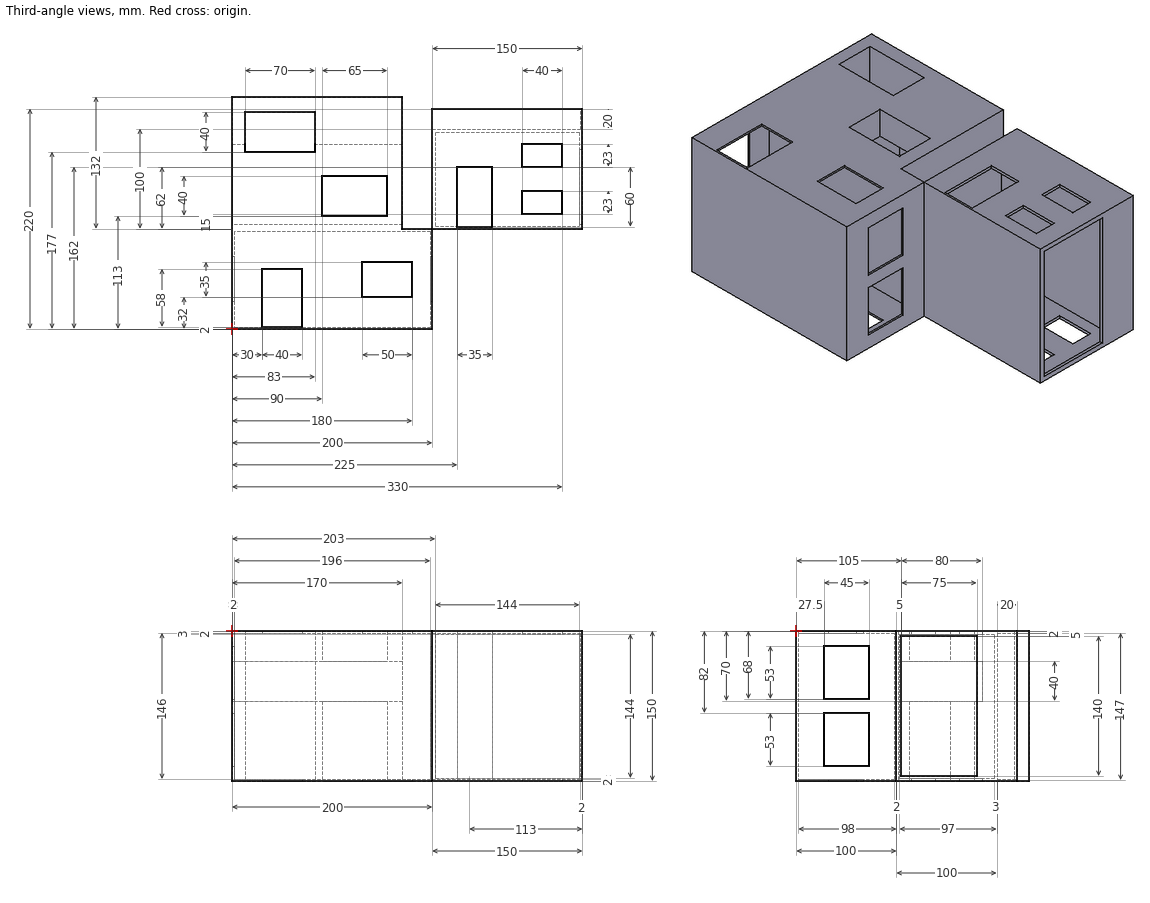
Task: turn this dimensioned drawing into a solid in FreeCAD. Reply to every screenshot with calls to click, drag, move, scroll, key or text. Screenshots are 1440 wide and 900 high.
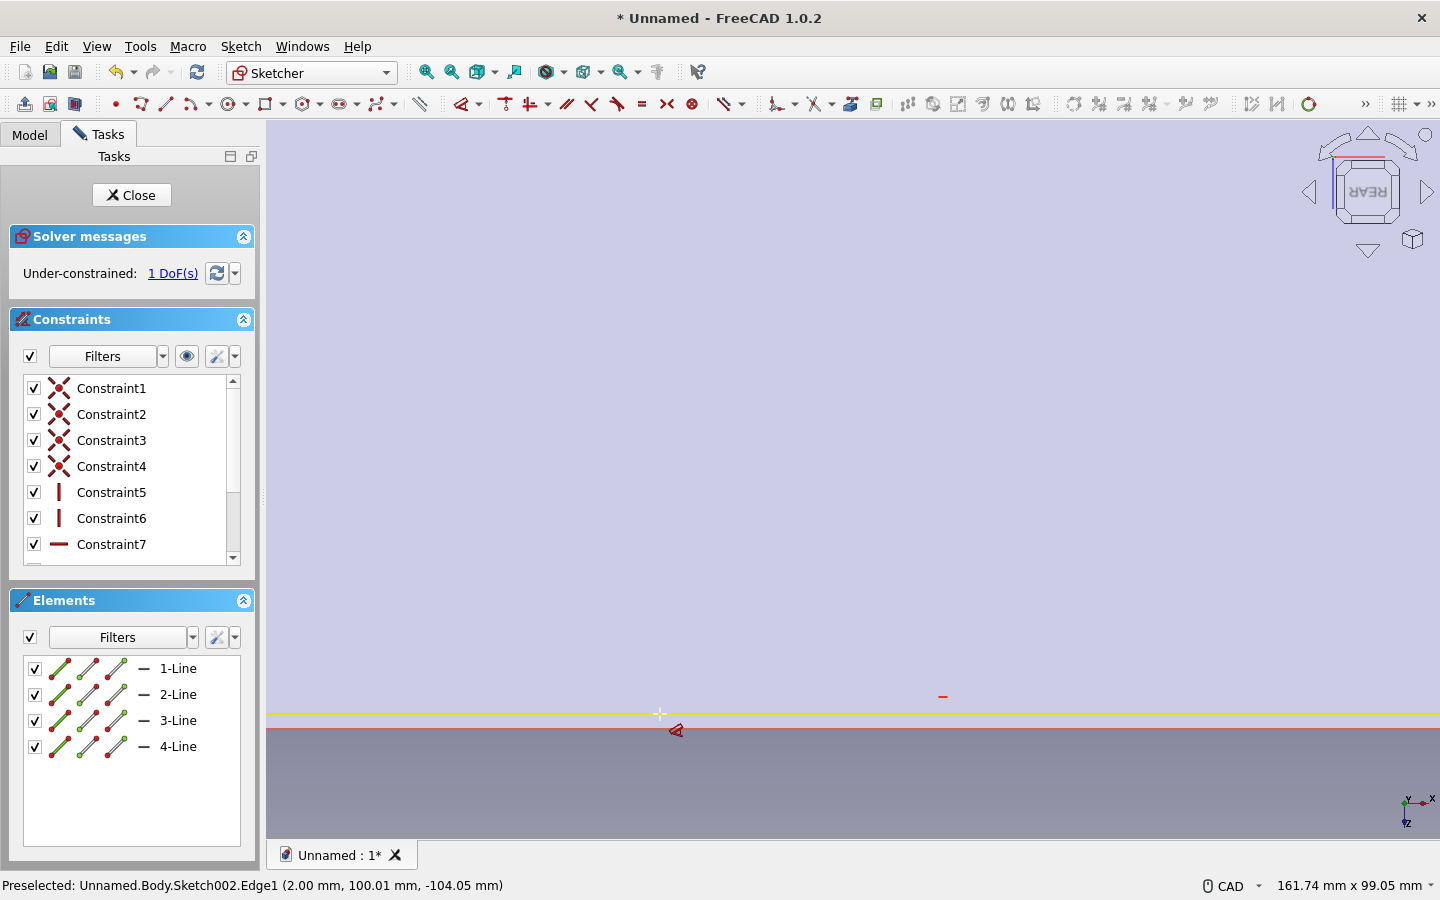
click(659, 714)
click(784, 748)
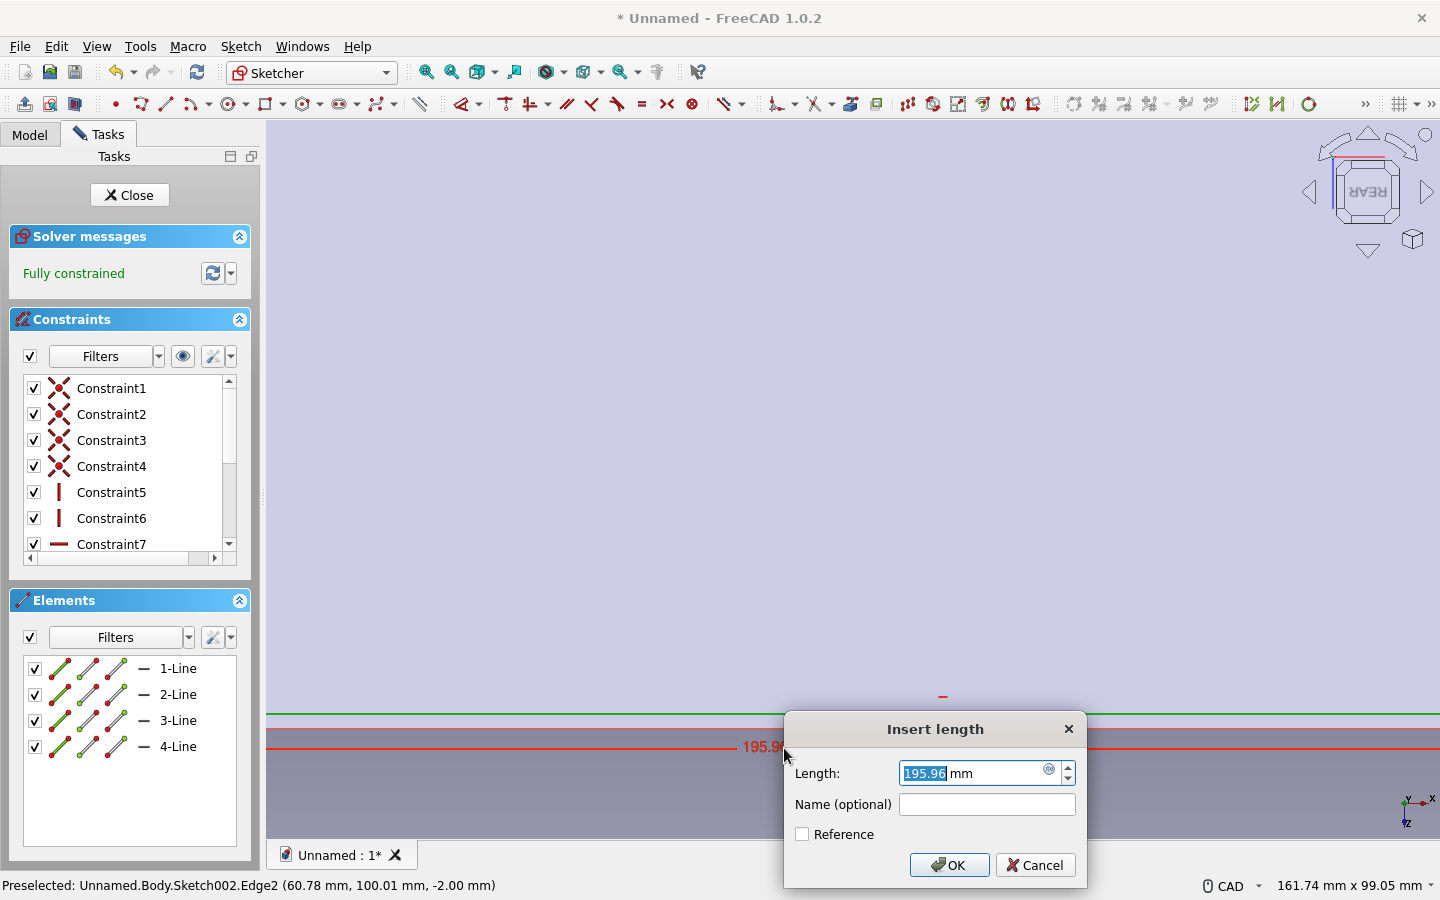
text(196)
key(Return)
key(Escape)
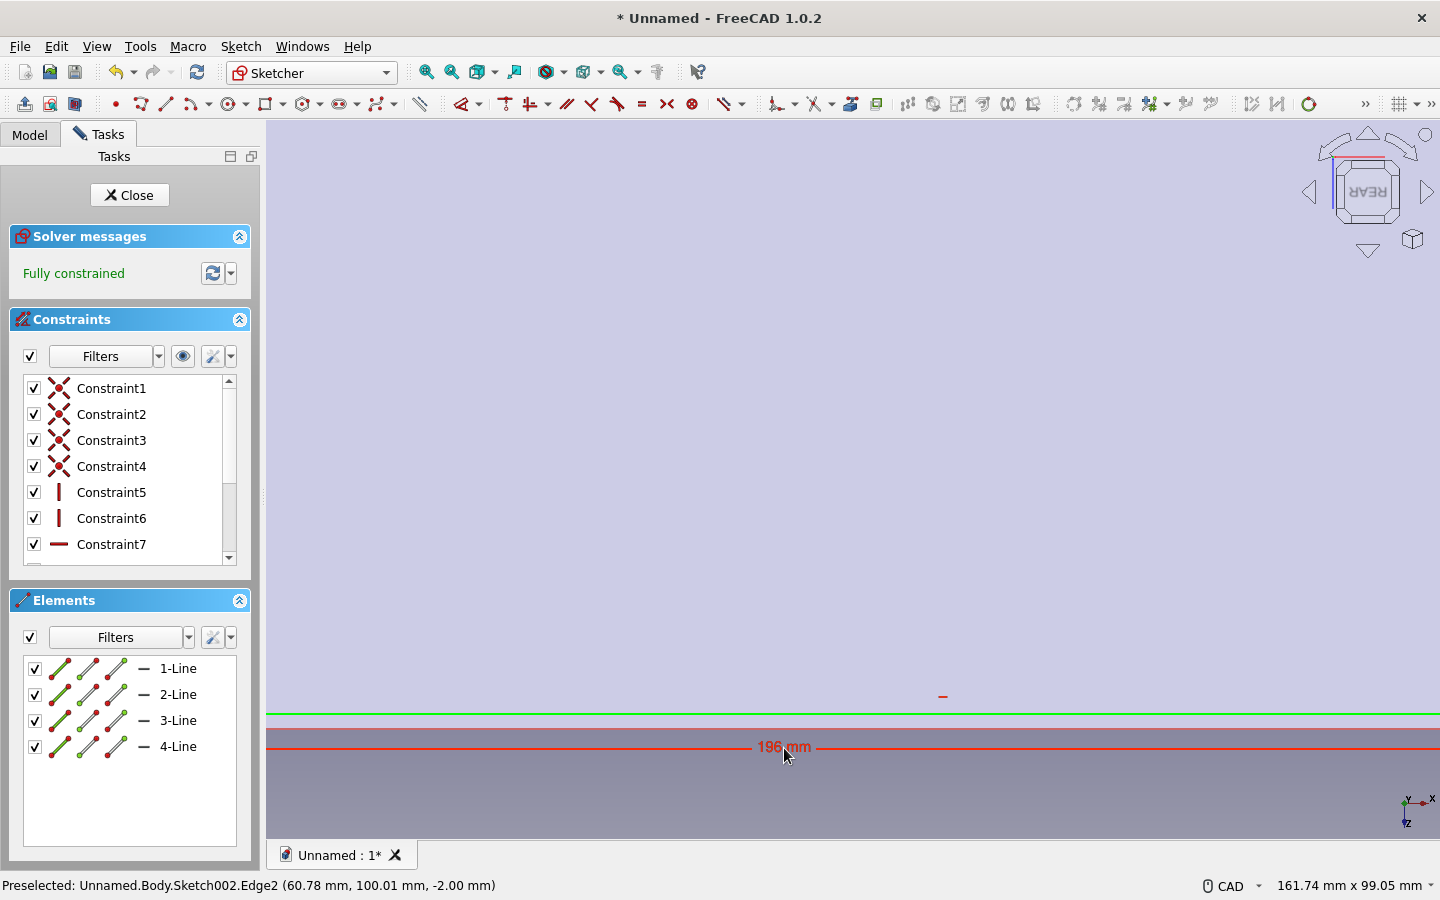
click(130, 195)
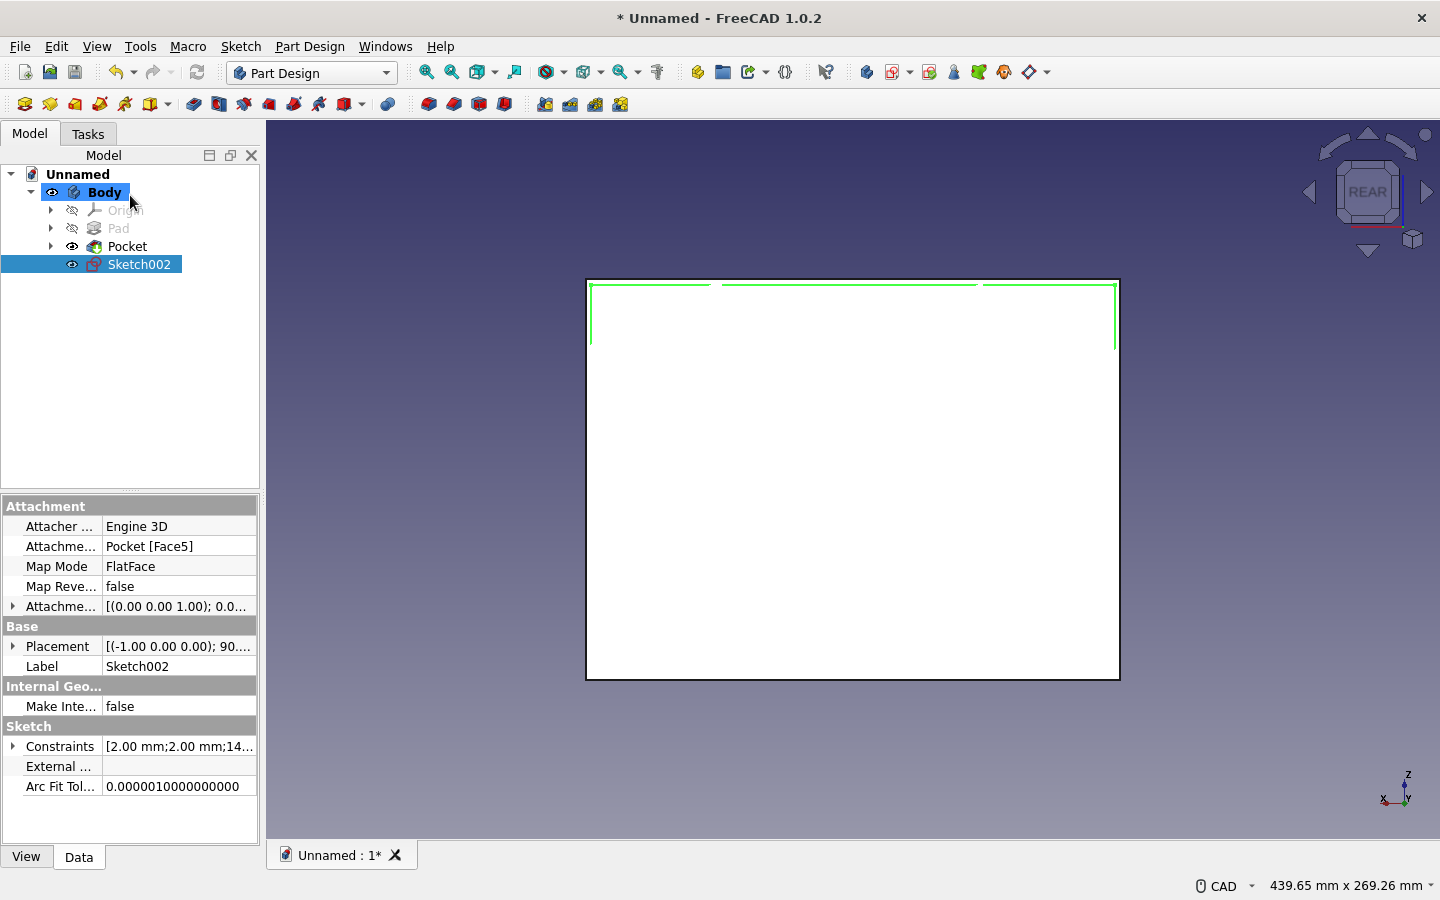
click(194, 104)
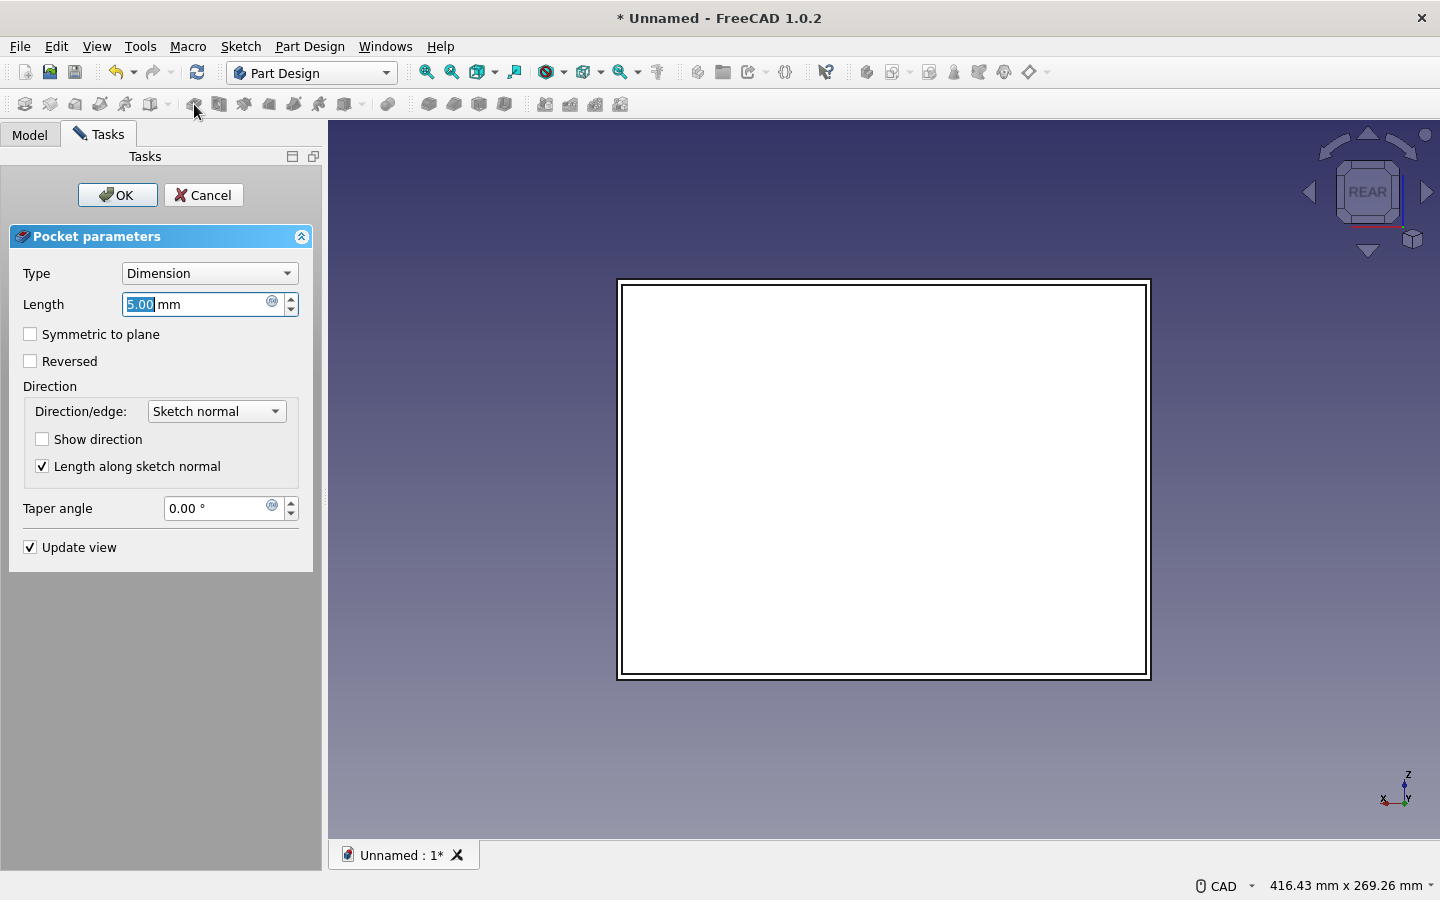
text(98)
key(Tab)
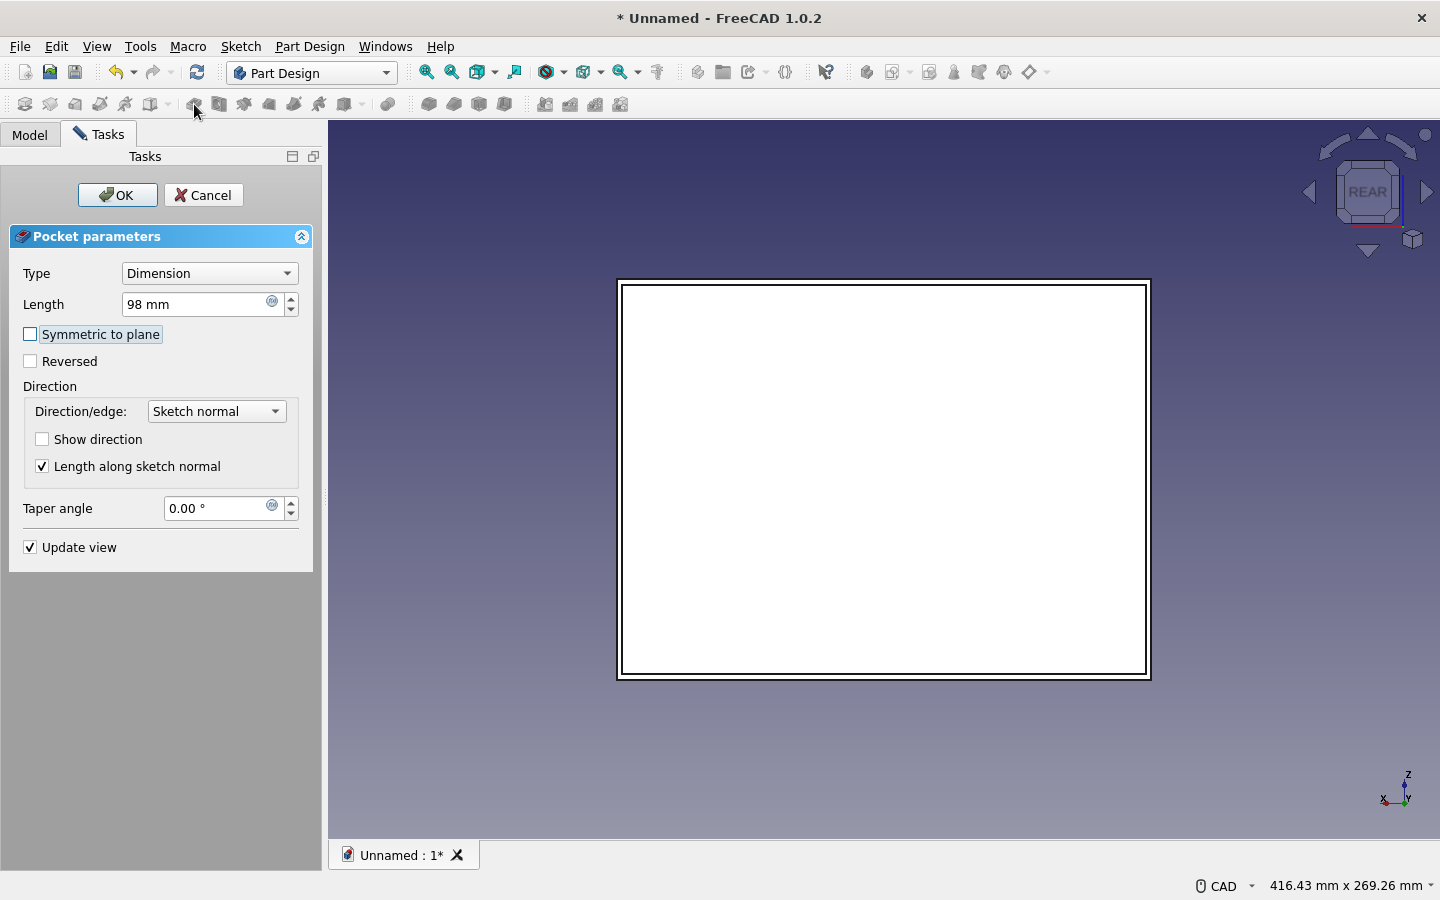
click(118, 195)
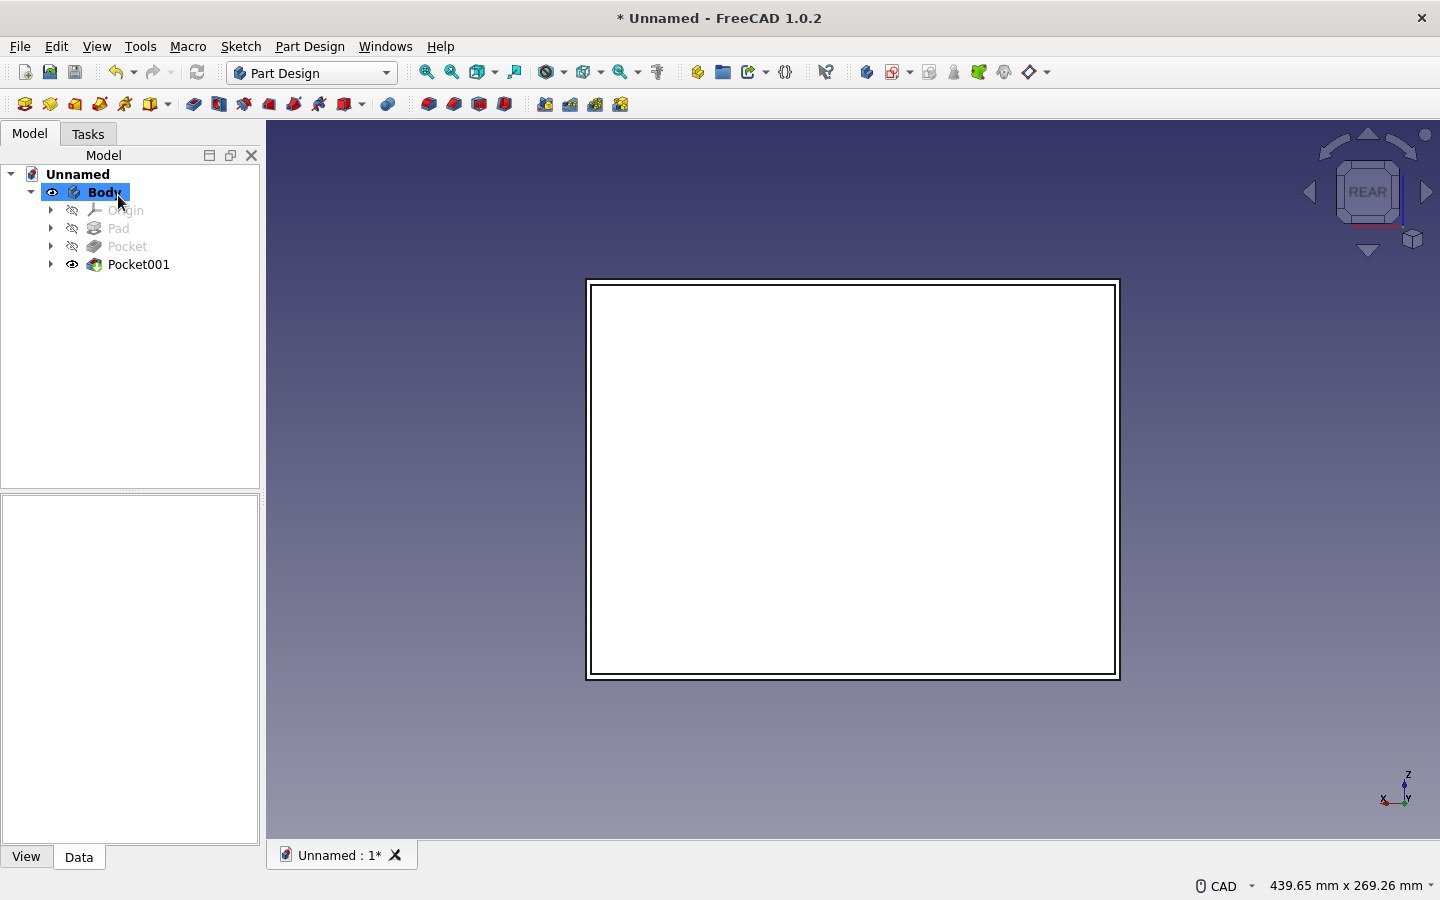
scroll(942, 675, up, 10)